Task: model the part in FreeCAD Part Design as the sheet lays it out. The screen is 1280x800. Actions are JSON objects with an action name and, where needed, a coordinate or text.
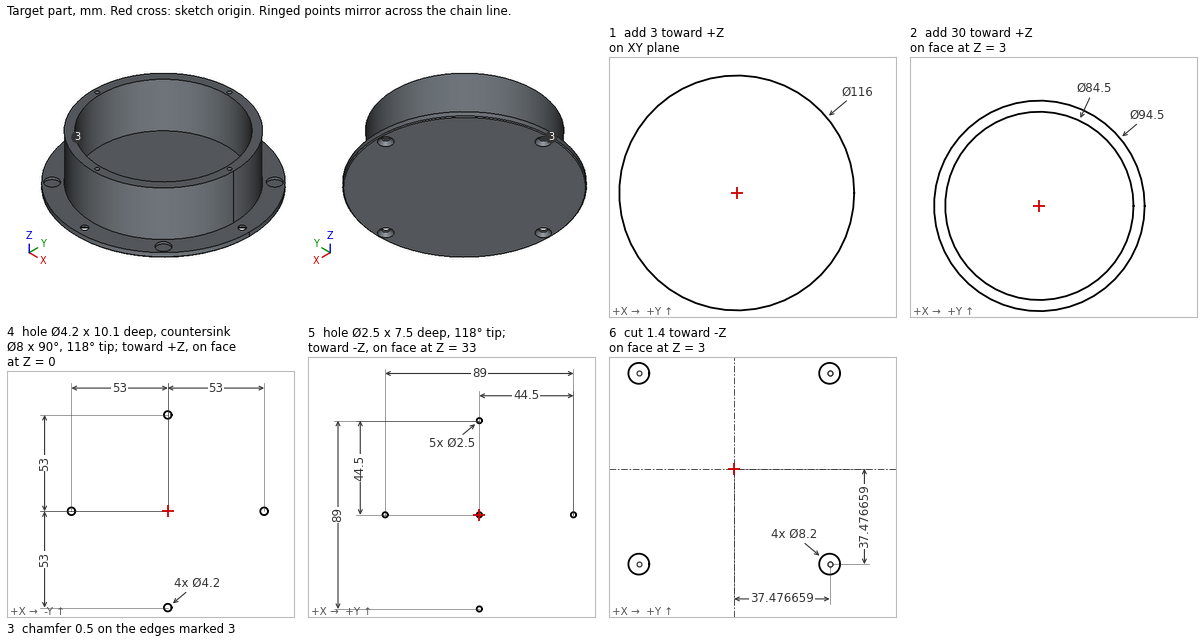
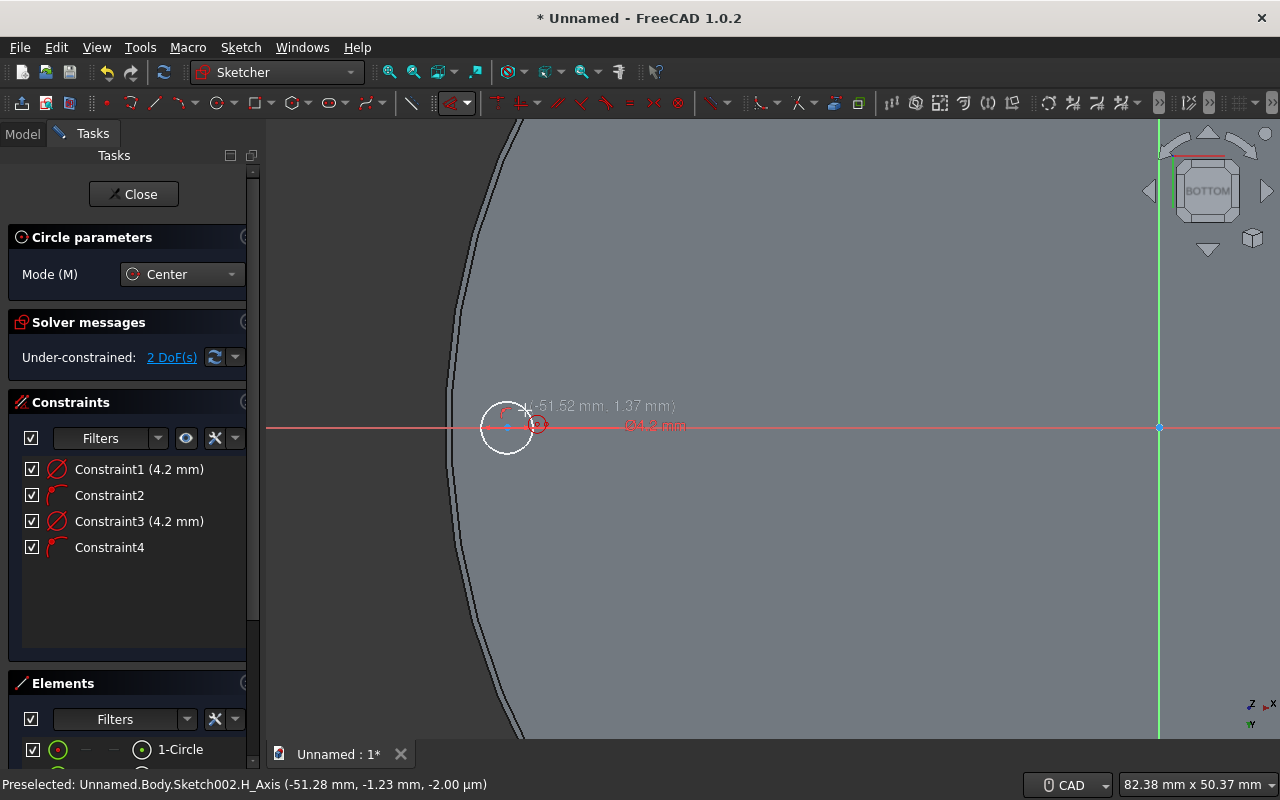
{"action": "scroll", "coordinate": [509, 430], "scroll_direction": "down", "scroll_amount": 6}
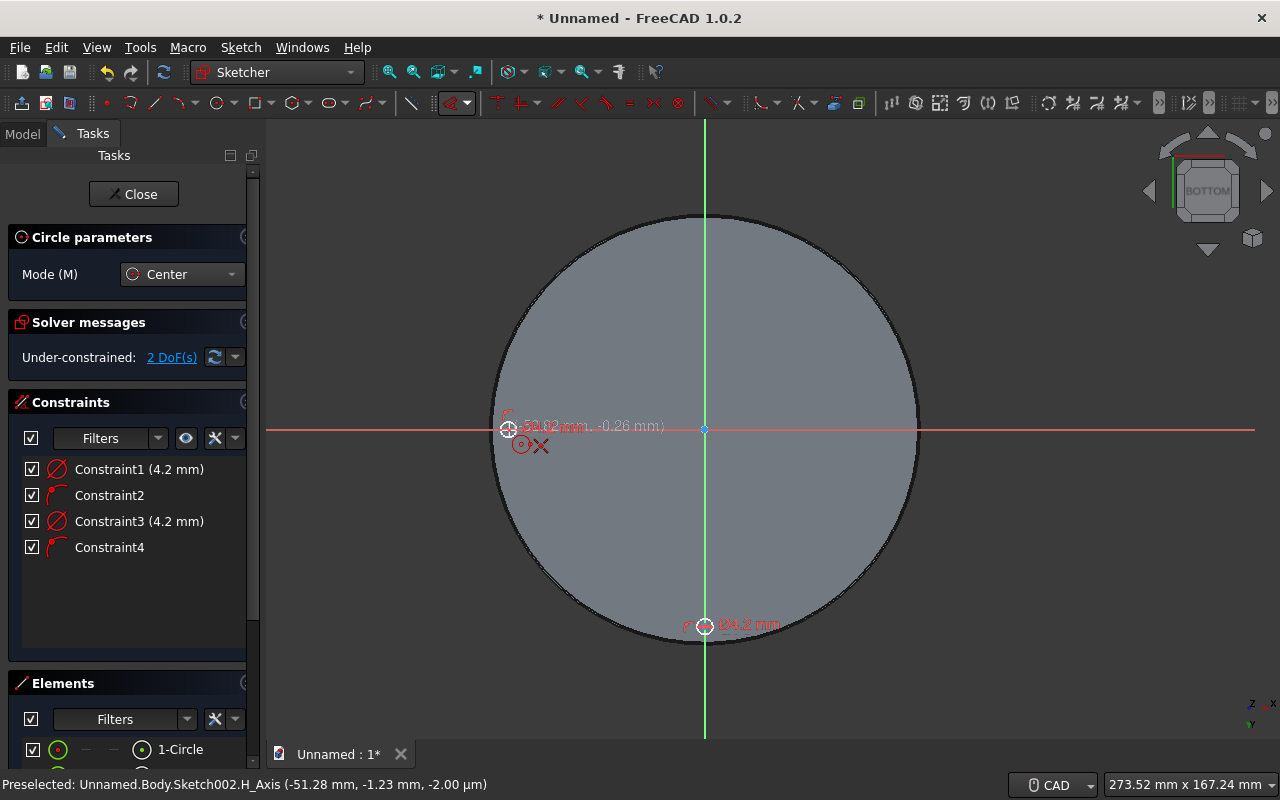
{"action": "scroll", "coordinate": [705, 233], "scroll_direction": "up", "scroll_amount": 6}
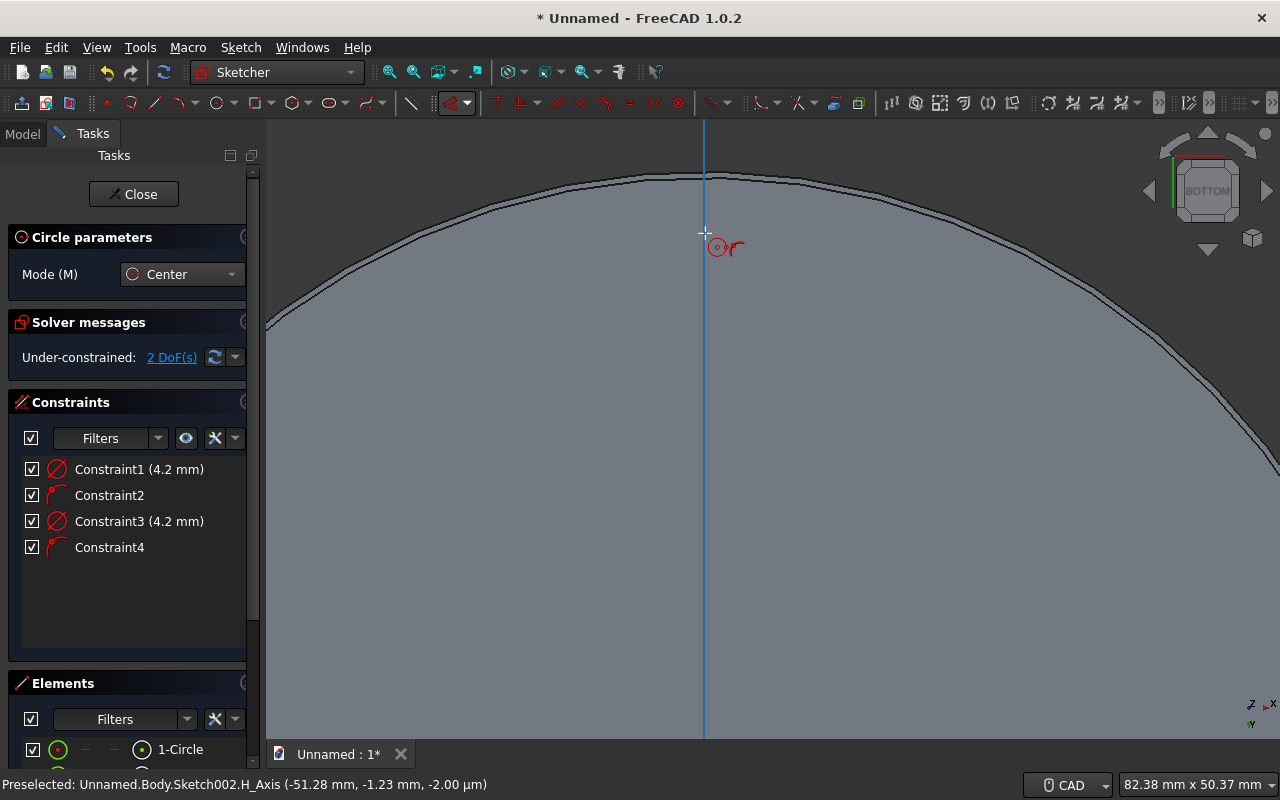
{"action": "left_click", "coordinate": [704, 233]}
{"action": "mouse_move", "coordinate": [722, 215]}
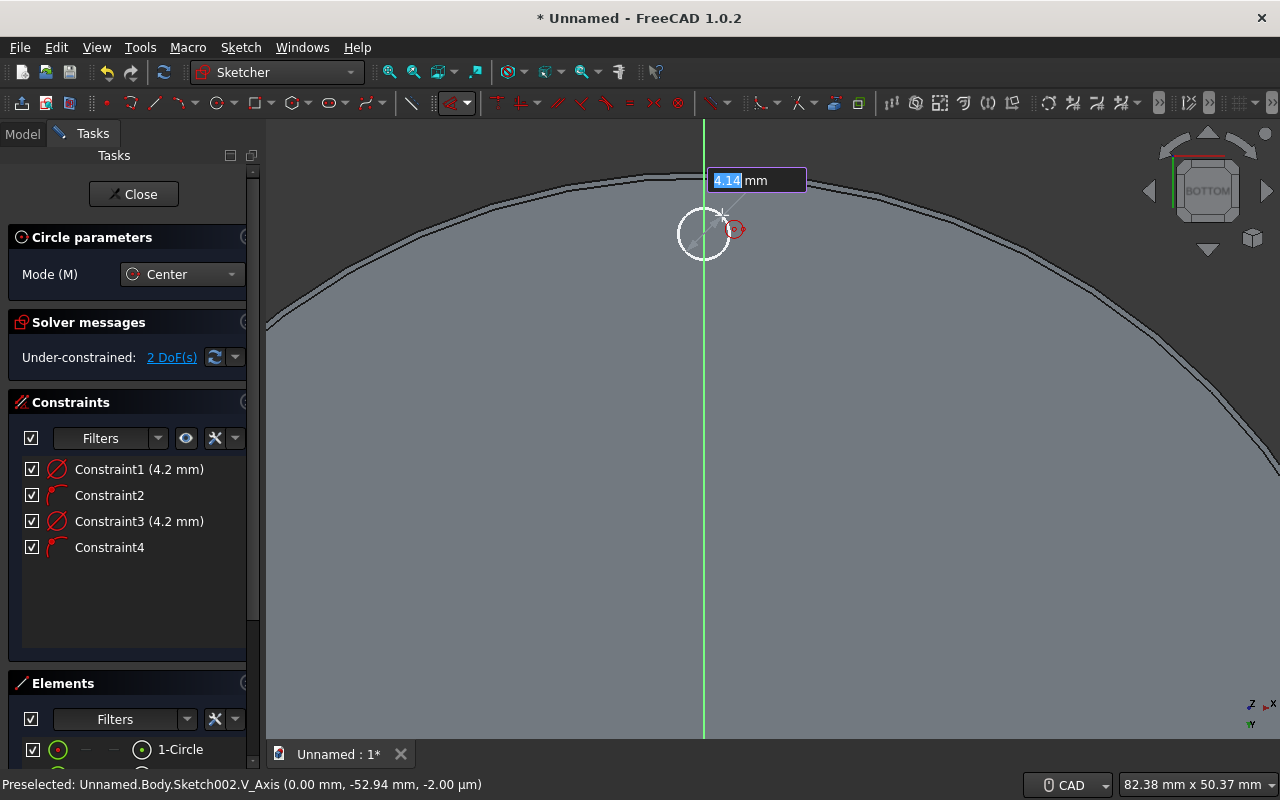
{"action": "type", "text": "4.2"}
{"action": "key", "text": "Return"}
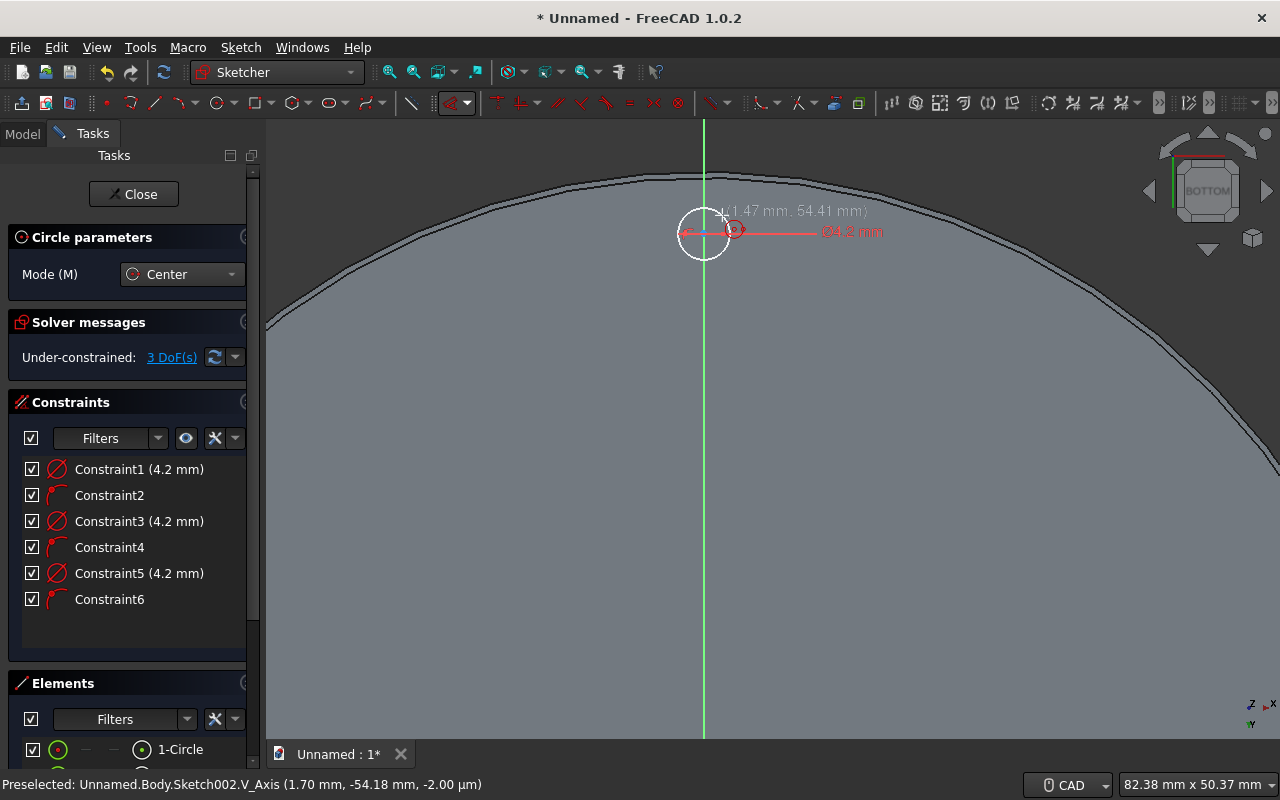
{"action": "scroll", "coordinate": [705, 232], "scroll_direction": "down", "scroll_amount": 6}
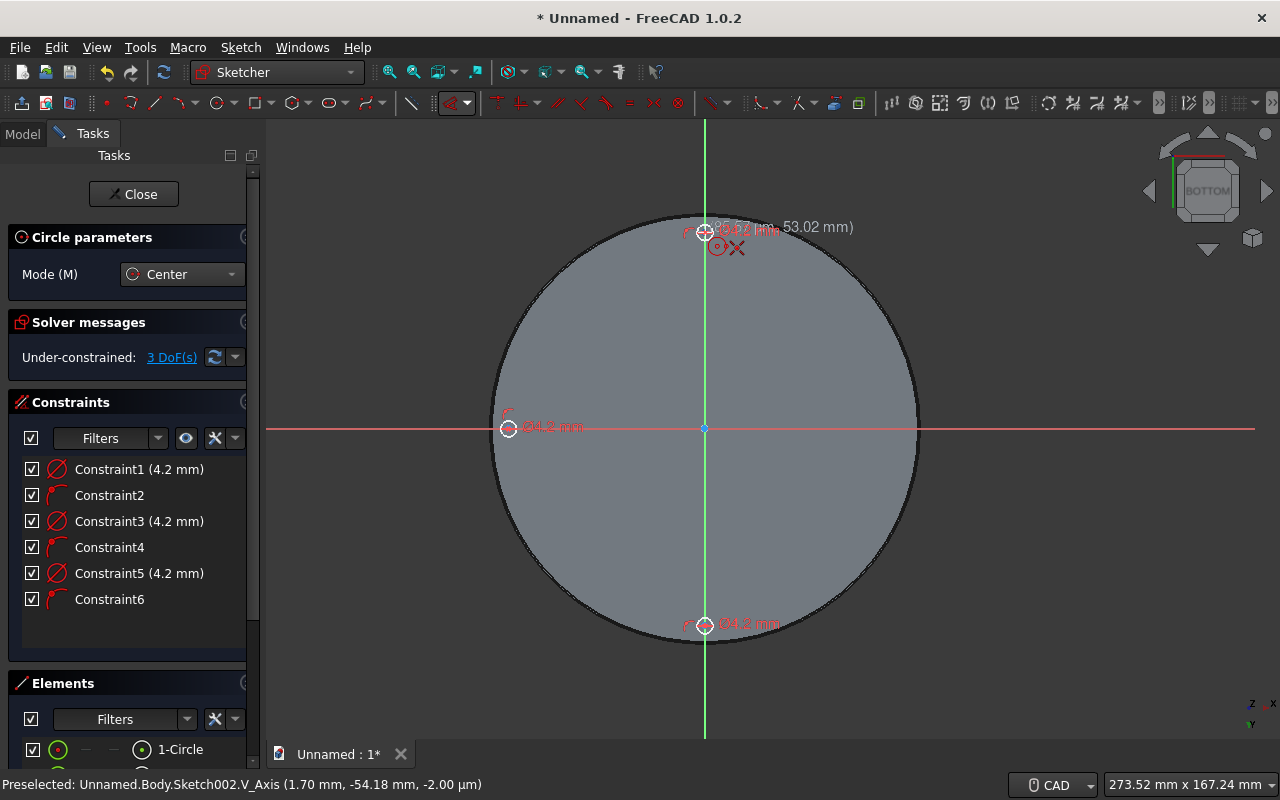
{"action": "scroll", "coordinate": [901, 429], "scroll_direction": "up", "scroll_amount": 6}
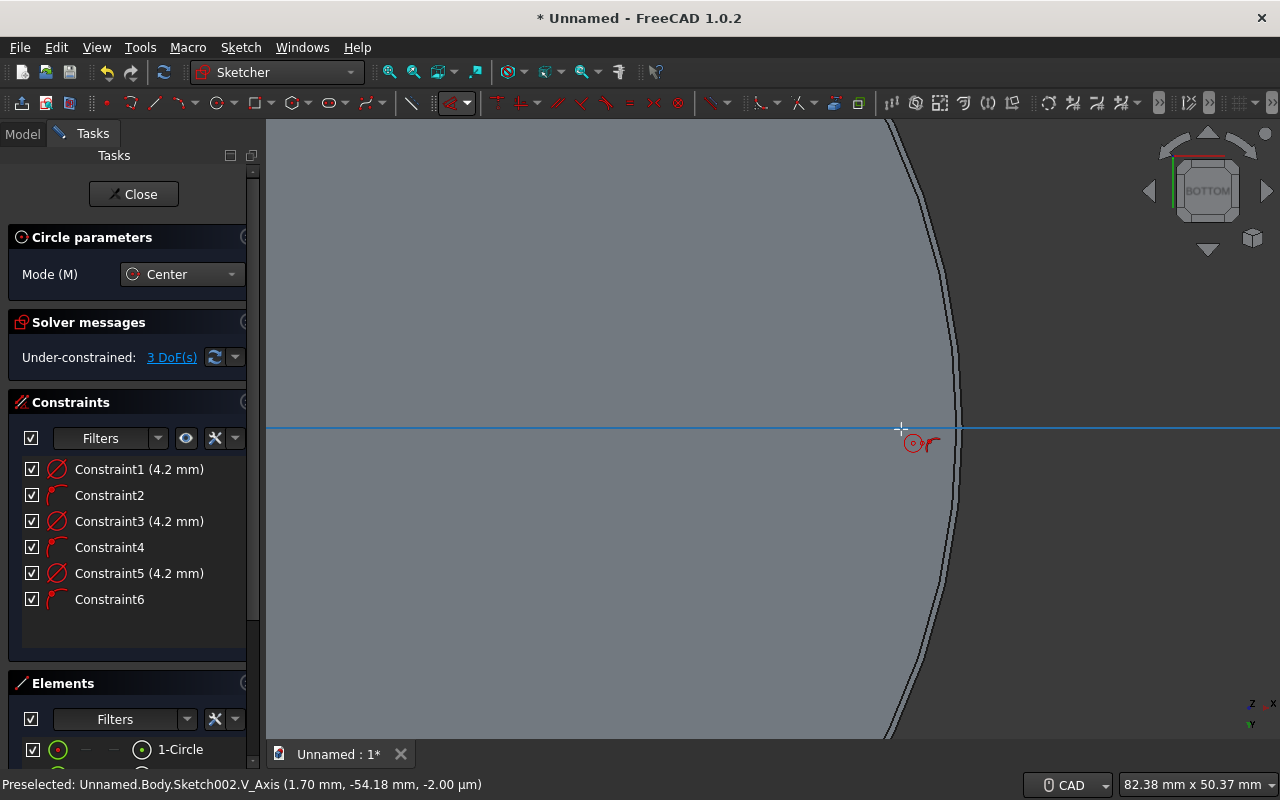
{"action": "left_click", "coordinate": [901, 428]}
{"action": "mouse_move", "coordinate": [919, 410]}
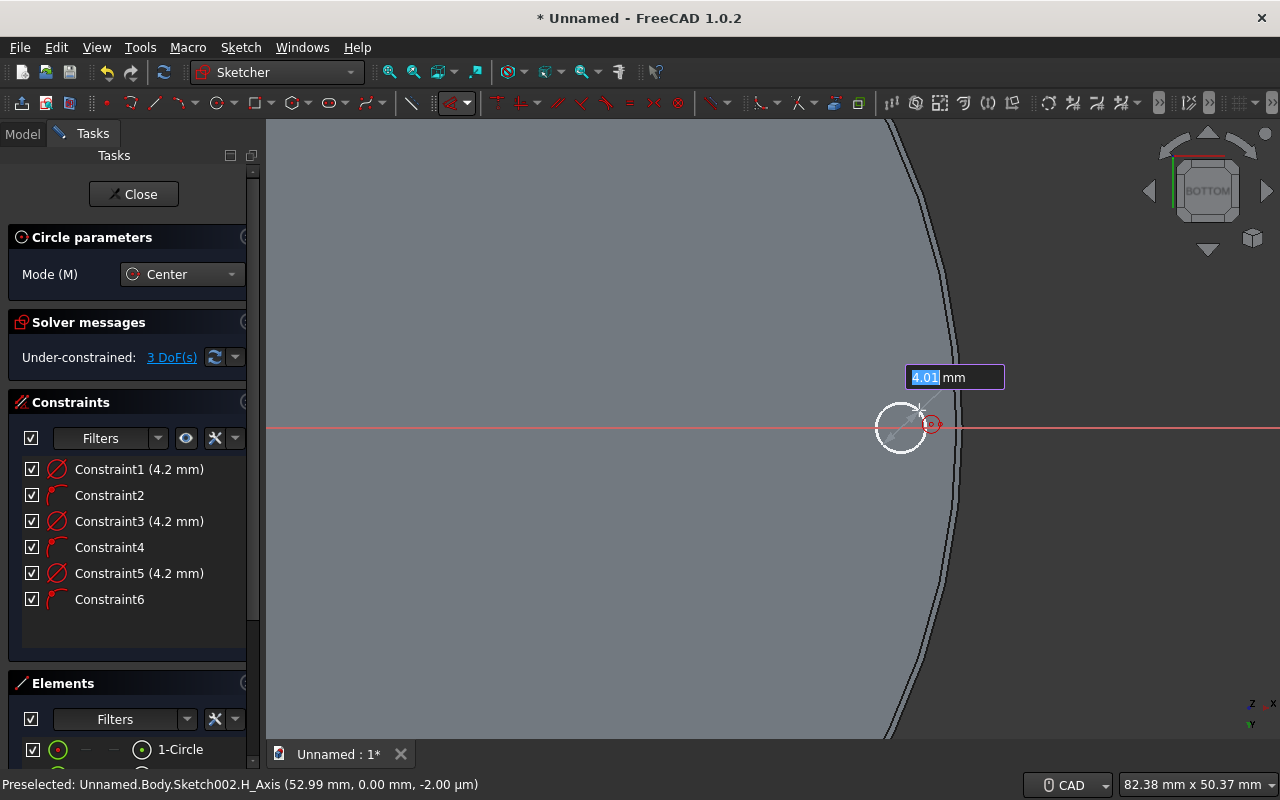
{"action": "type", "text": "4.2"}
{"action": "key", "text": "Return"}
{"action": "key", "text": "Escape"}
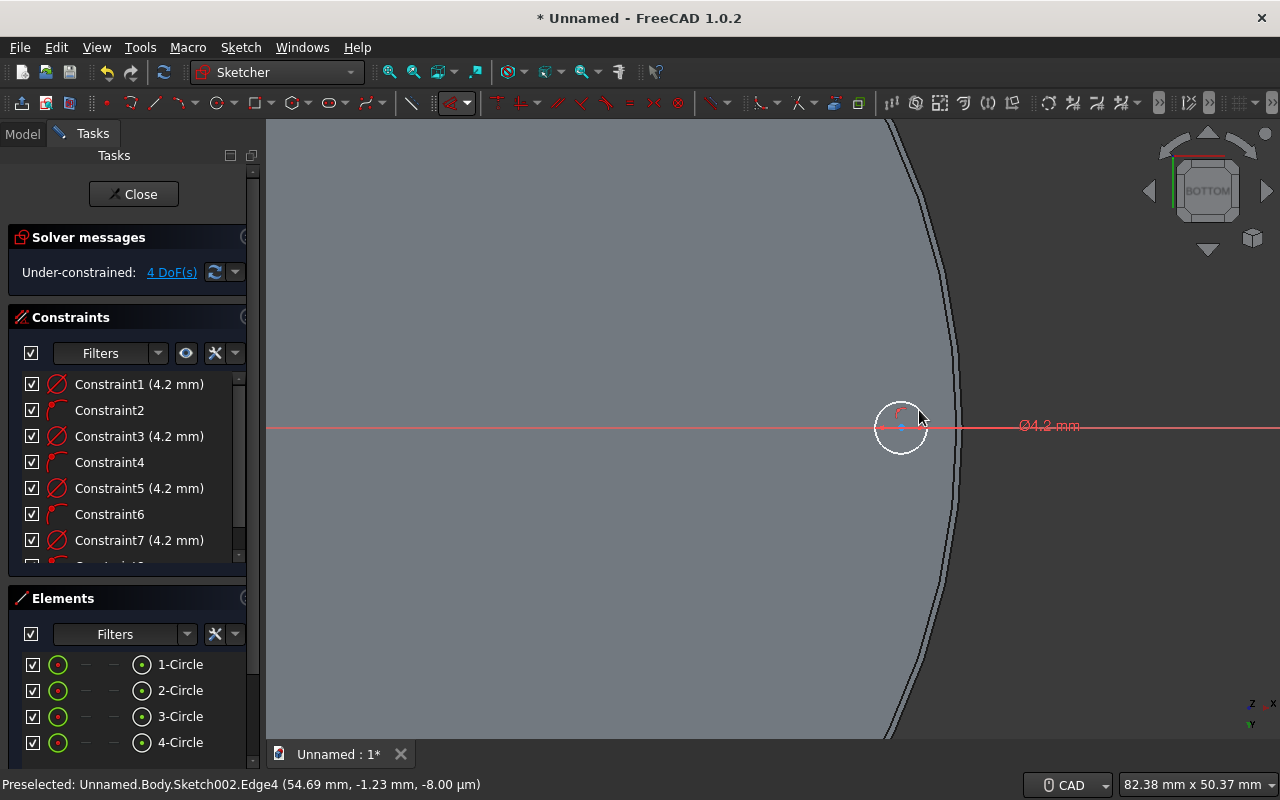
{"action": "left_click", "coordinate": [450, 104]}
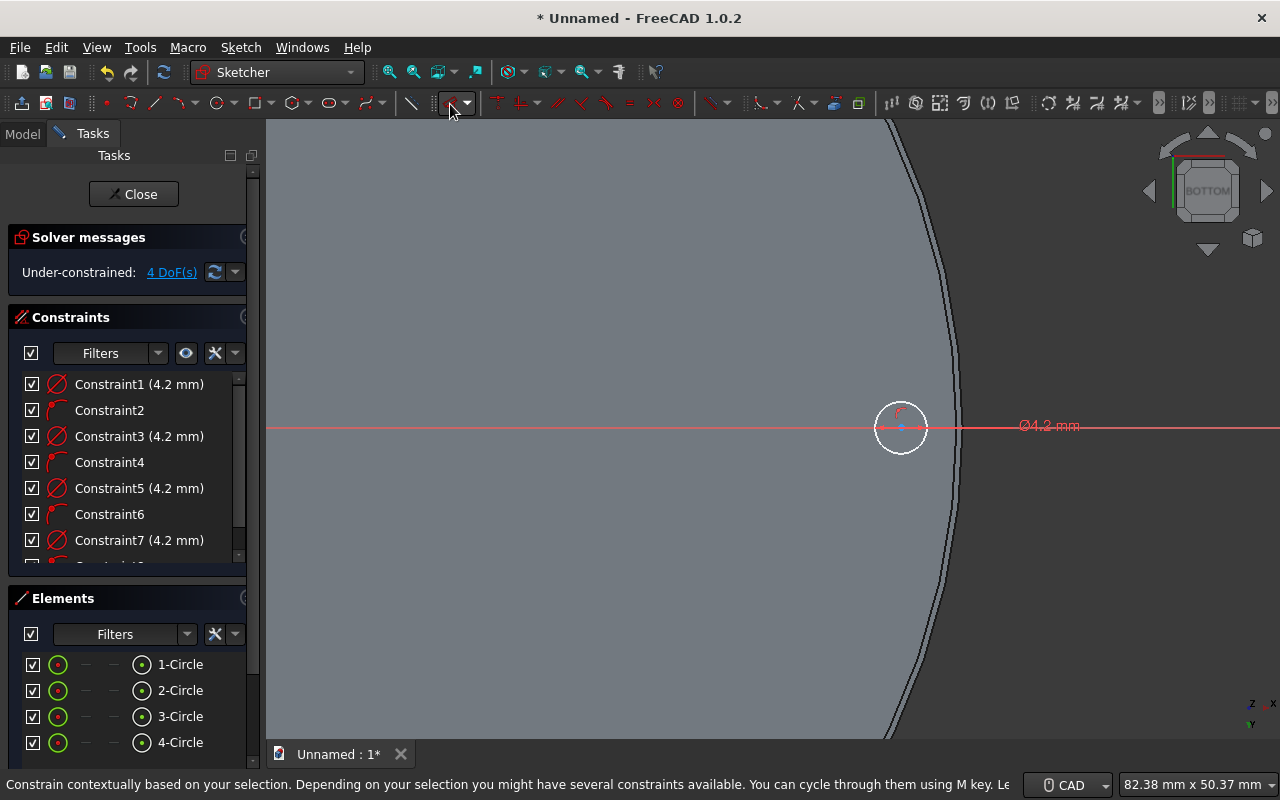
{"action": "scroll", "coordinate": [901, 430], "scroll_direction": "down", "scroll_amount": 6}